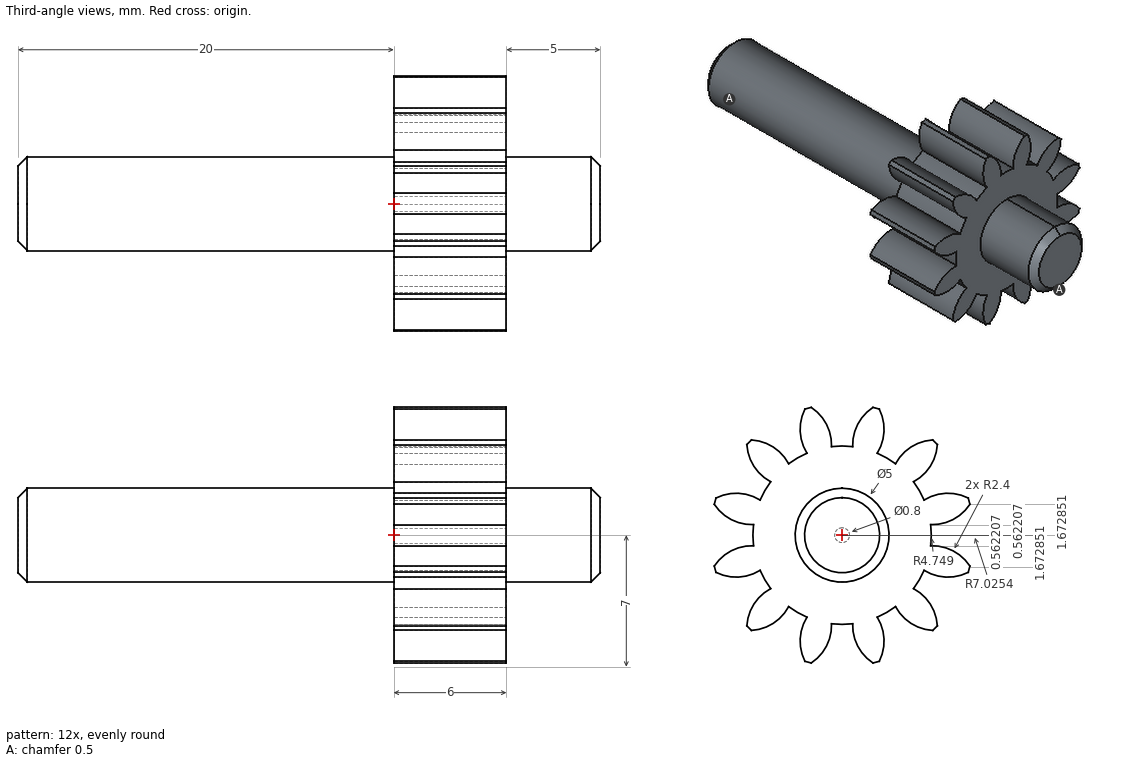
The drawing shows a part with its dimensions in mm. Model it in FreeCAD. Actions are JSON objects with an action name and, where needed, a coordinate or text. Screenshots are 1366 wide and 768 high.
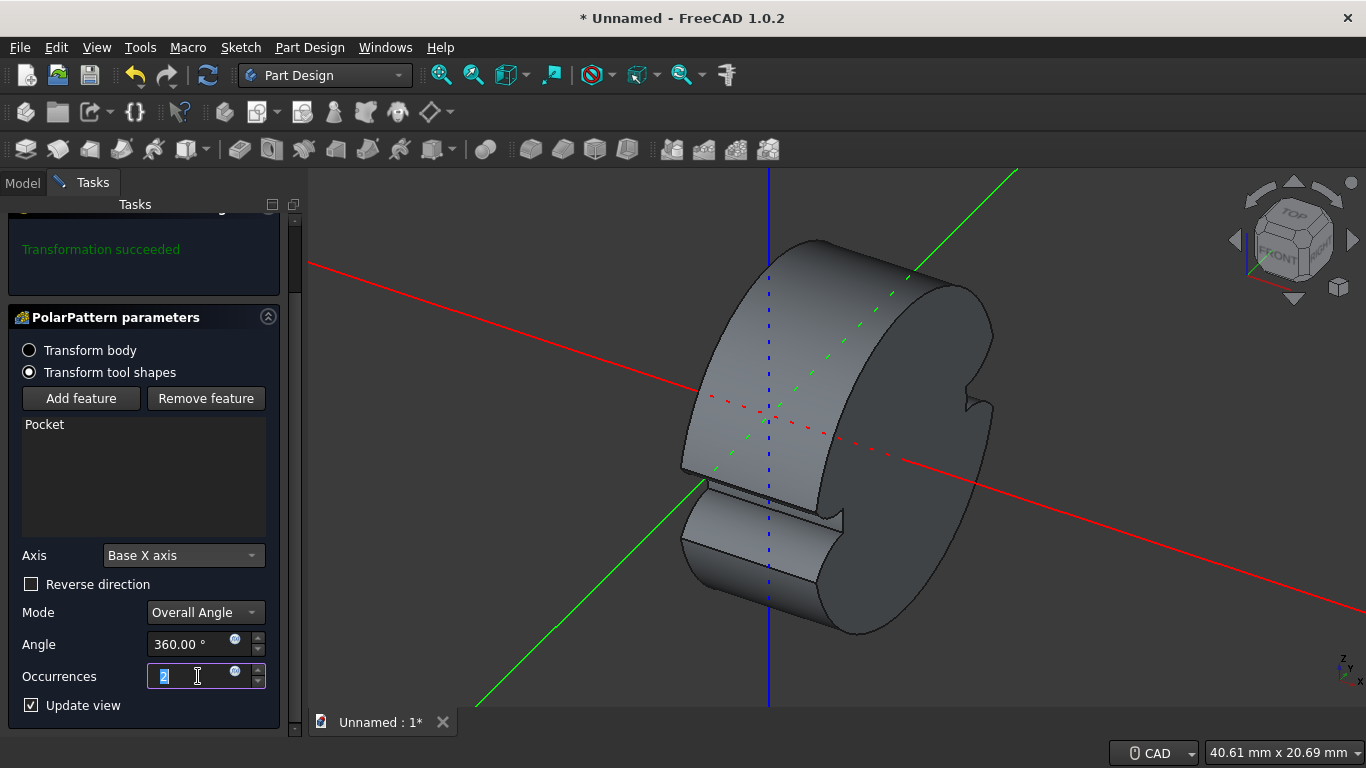
{"action": "type", "text": "12"}
{"action": "key", "text": "Tab"}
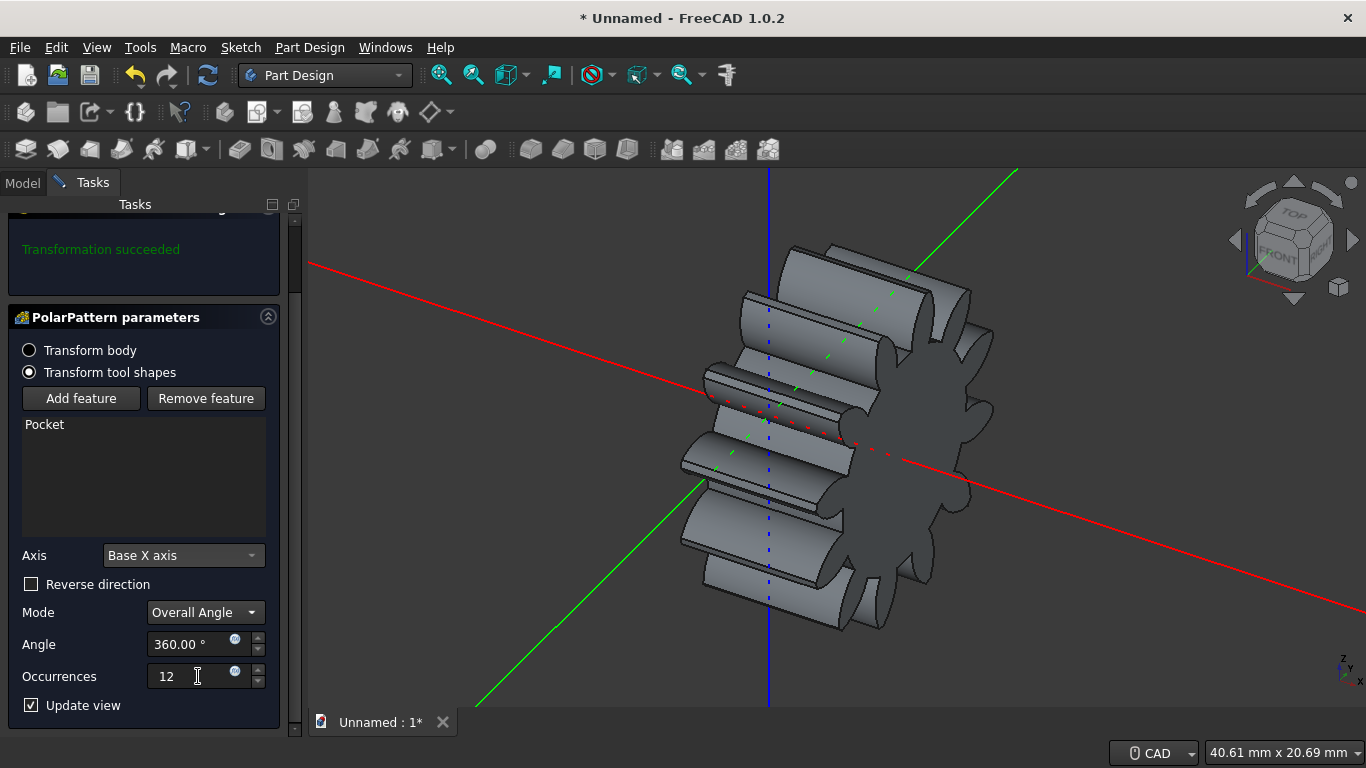
{"action": "scroll", "coordinate": [295, 475], "scroll_direction": "up", "scroll_amount": 3}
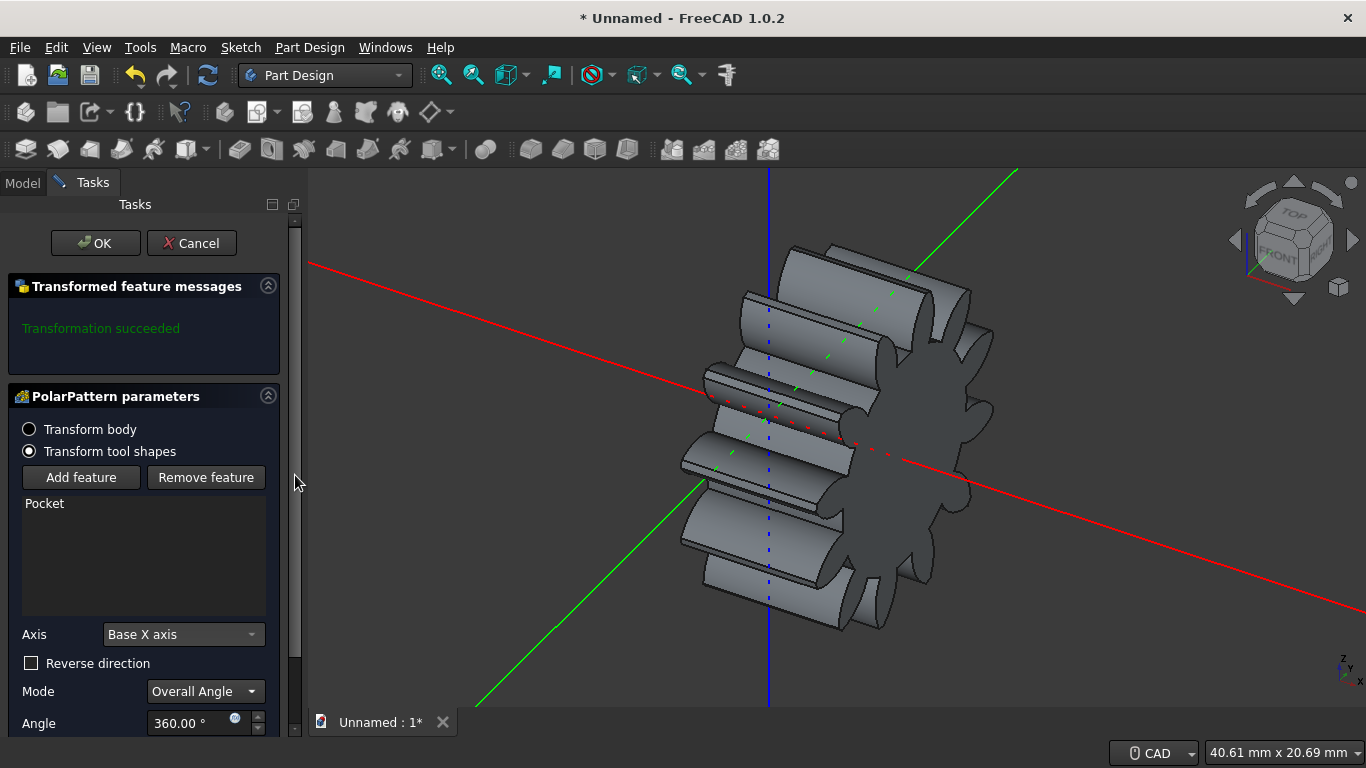
{"action": "left_click", "coordinate": [96, 243]}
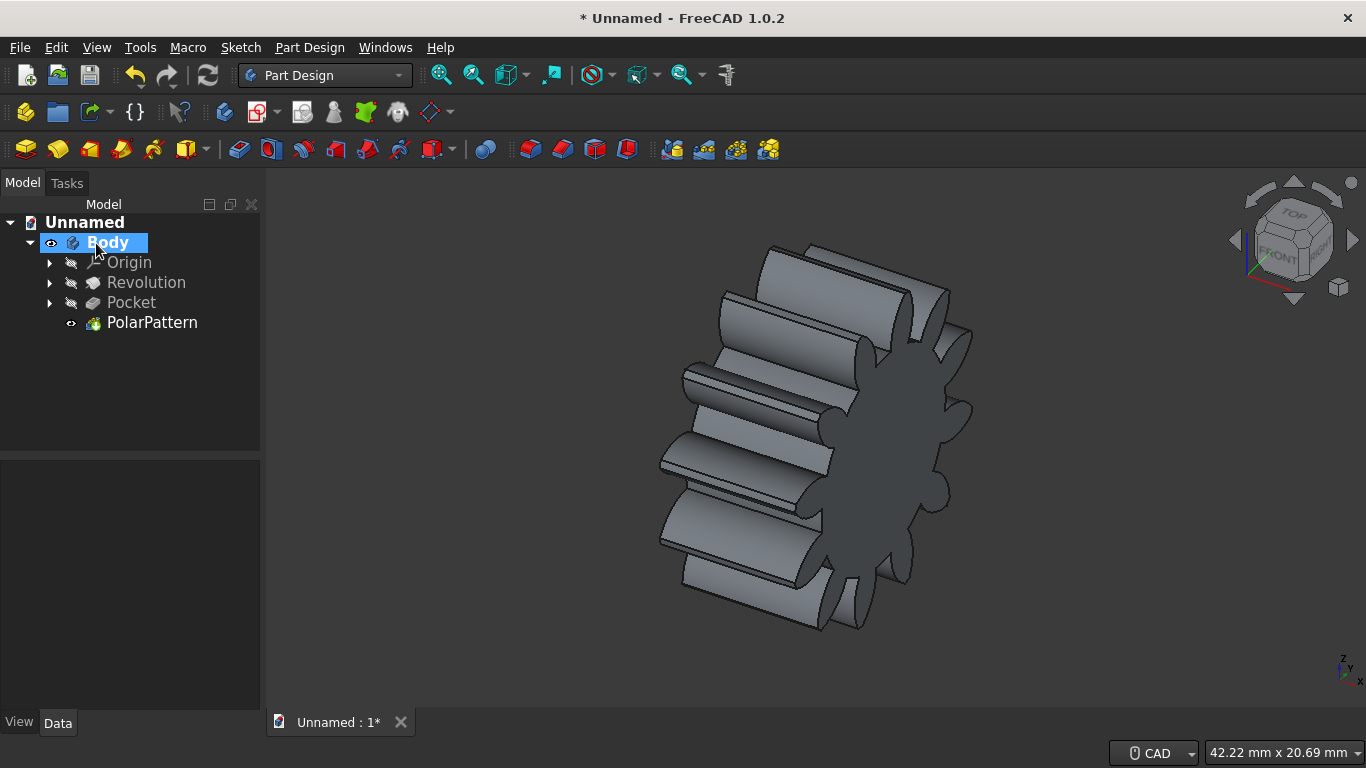
{"action": "left_click", "coordinate": [258, 112]}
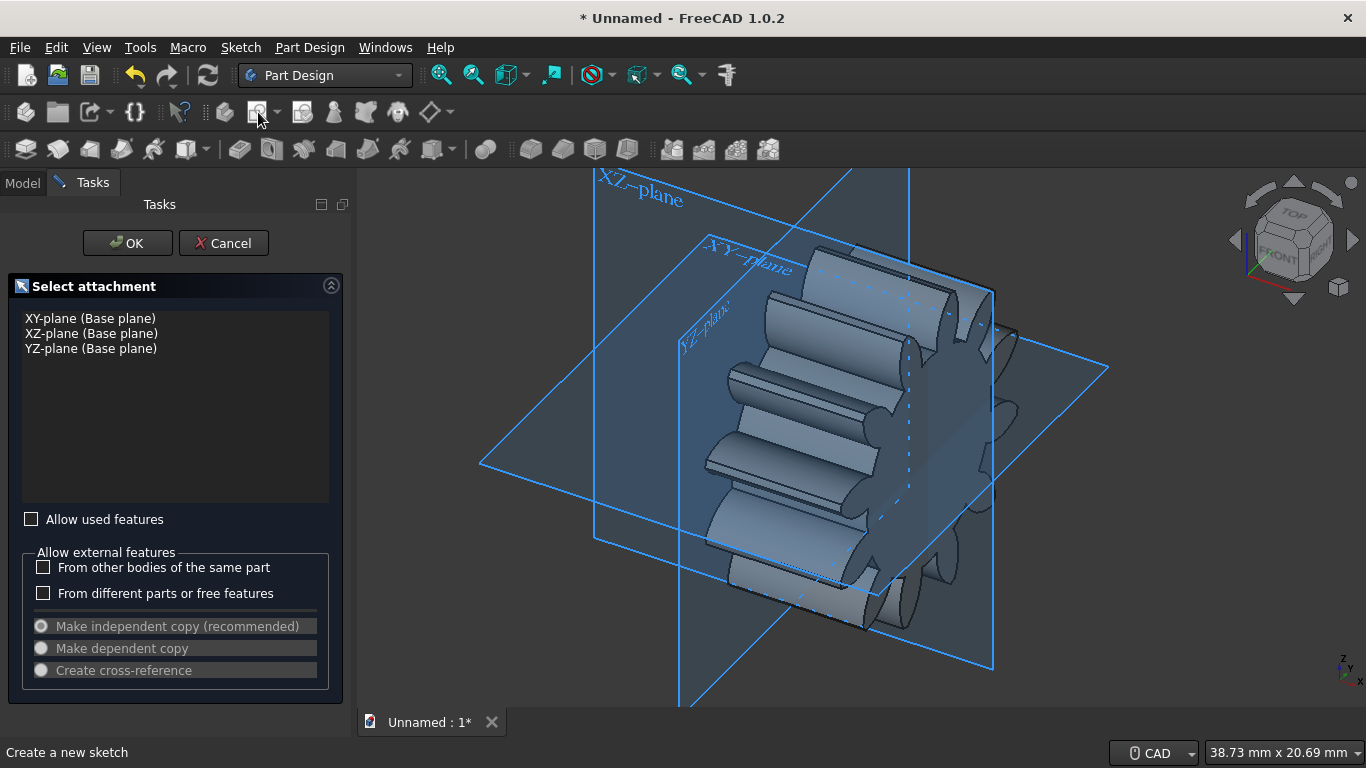
{"action": "left_click", "coordinate": [82, 348]}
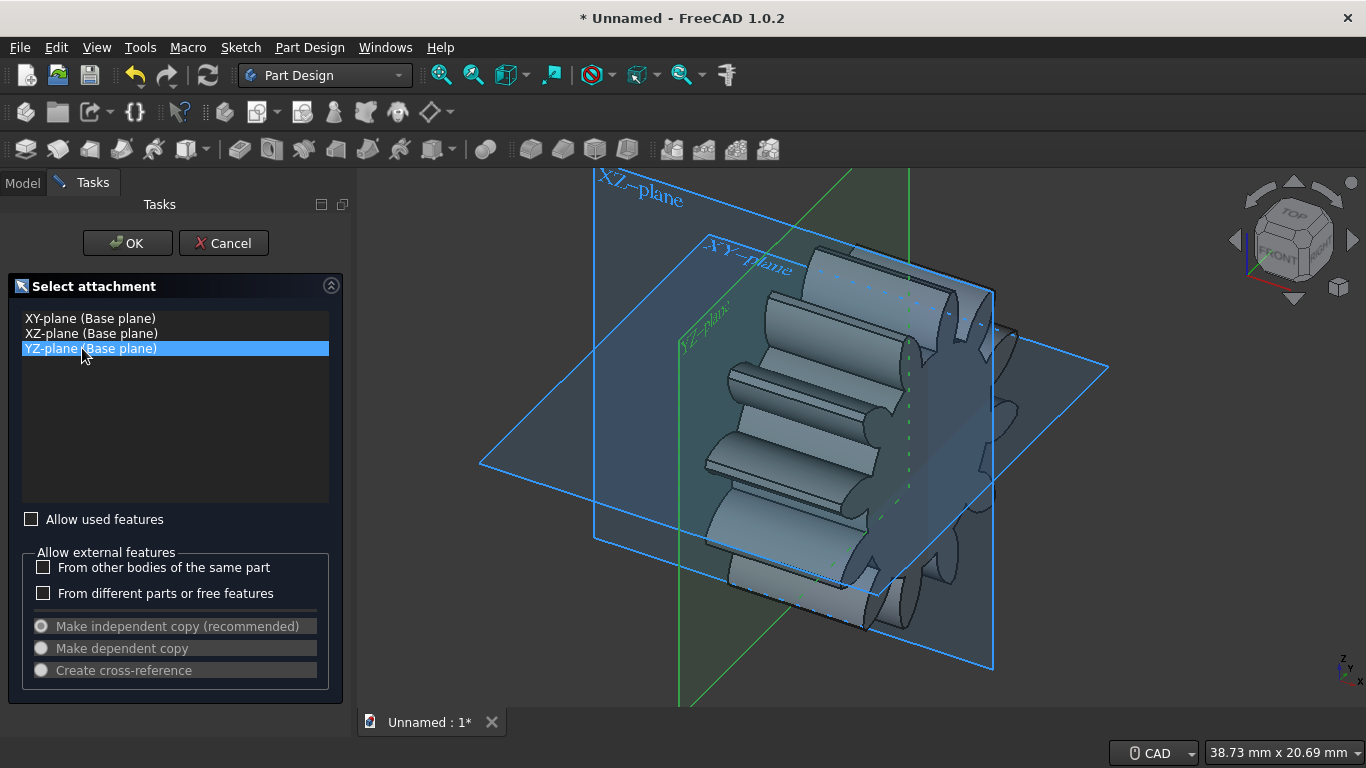
{"action": "left_click", "coordinate": [128, 243]}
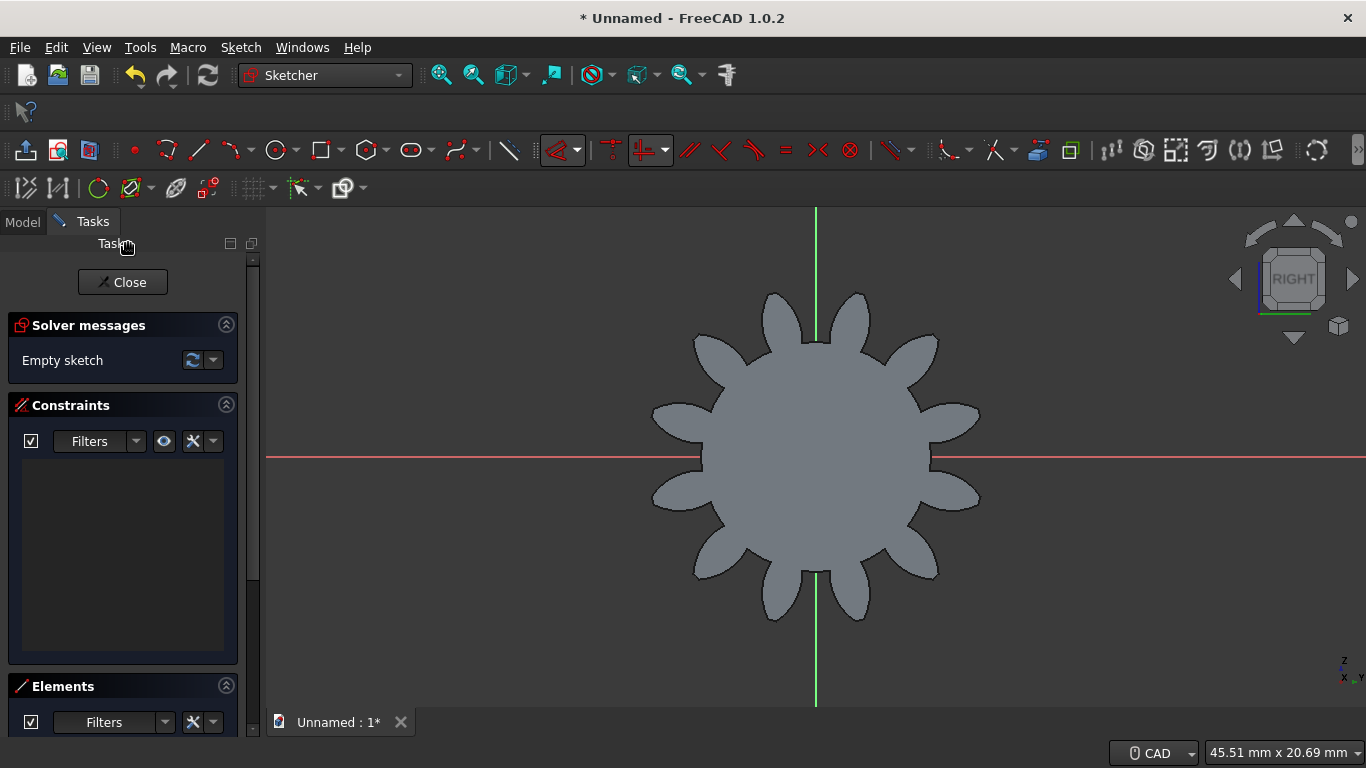
{"action": "left_click", "coordinate": [90, 150]}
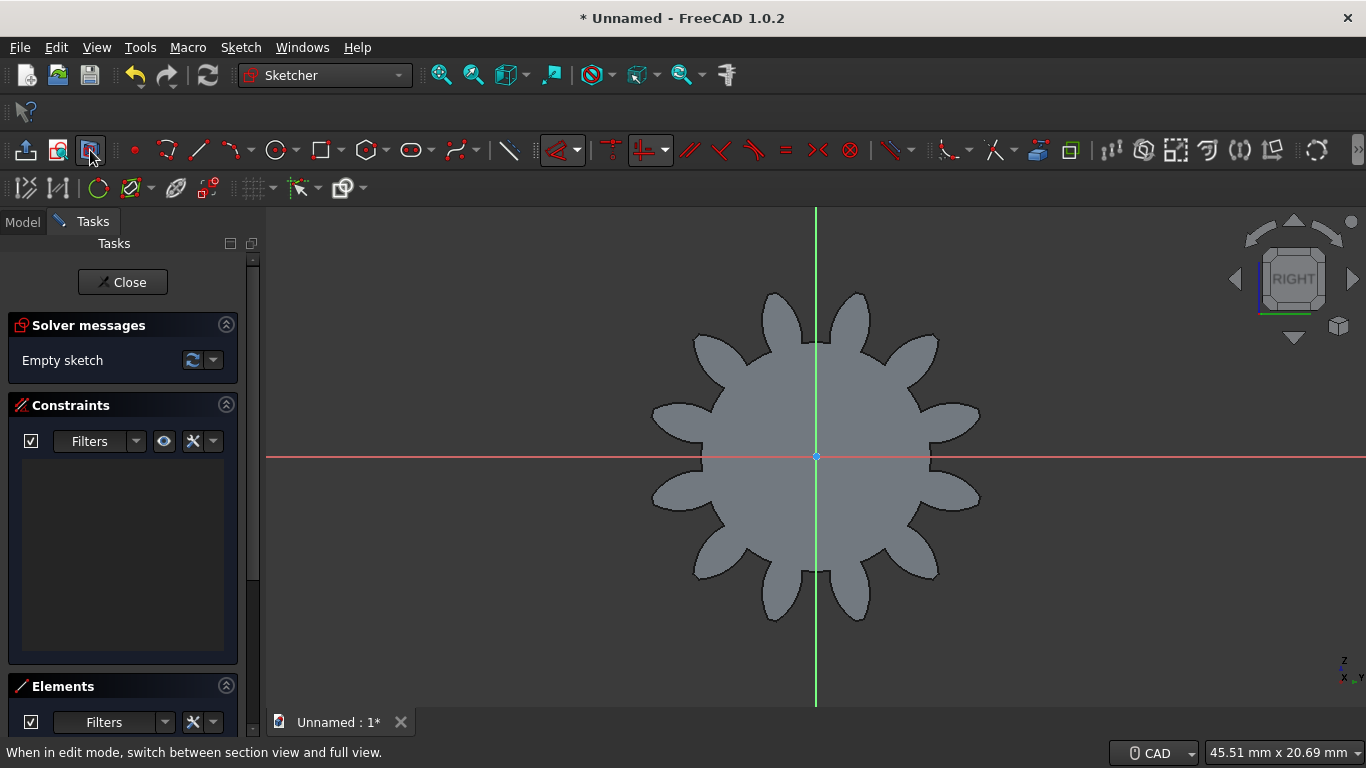
{"action": "scroll", "coordinate": [820, 457], "scroll_direction": "up", "scroll_amount": 14}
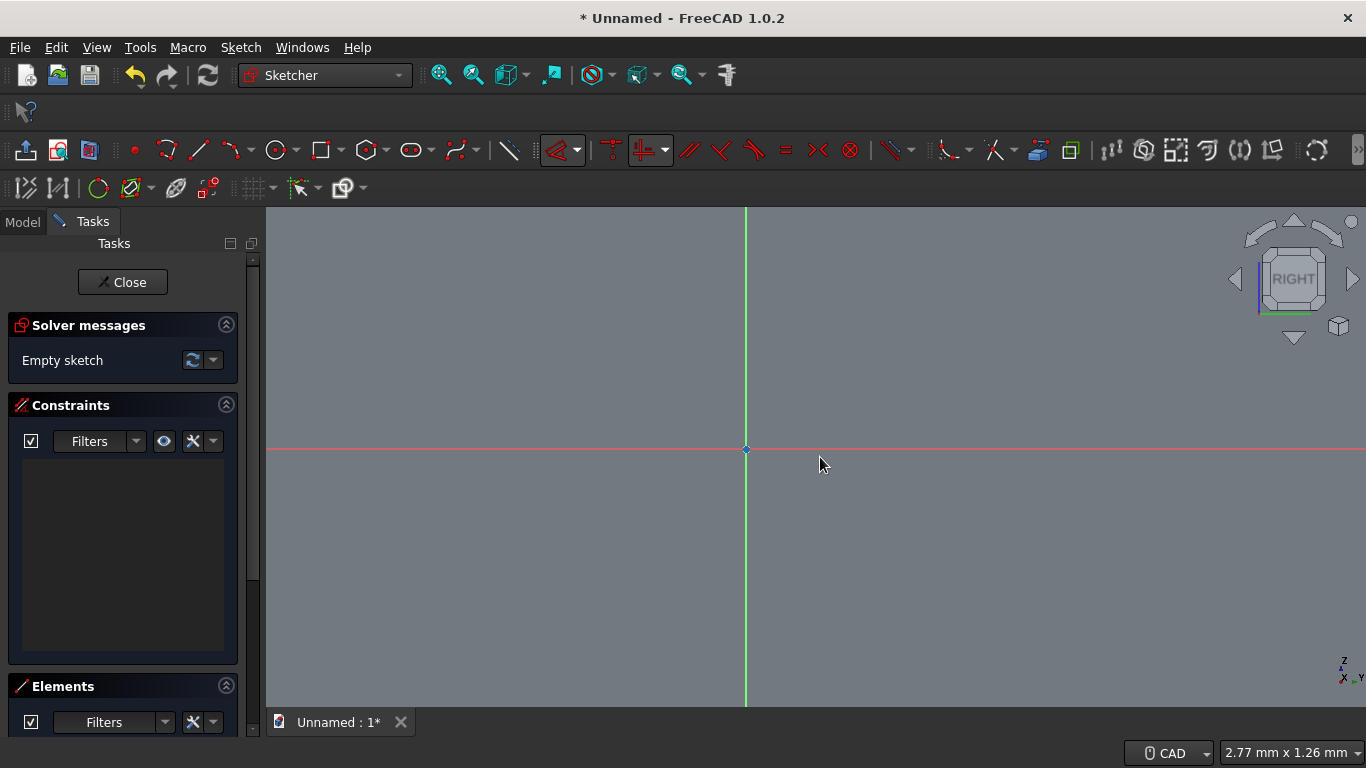
{"action": "left_click", "coordinate": [276, 150]}